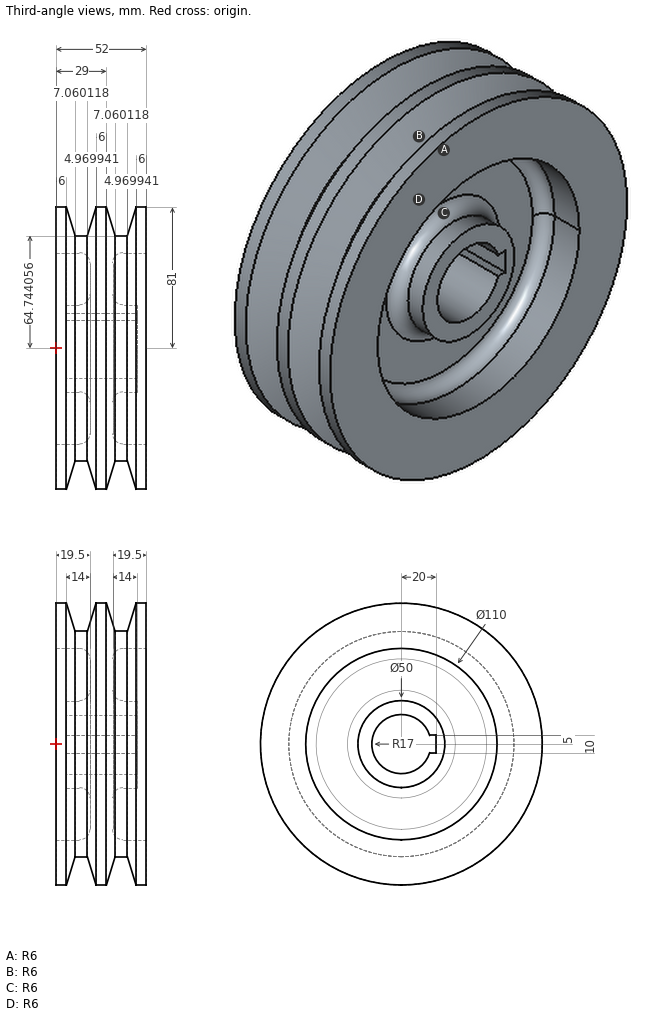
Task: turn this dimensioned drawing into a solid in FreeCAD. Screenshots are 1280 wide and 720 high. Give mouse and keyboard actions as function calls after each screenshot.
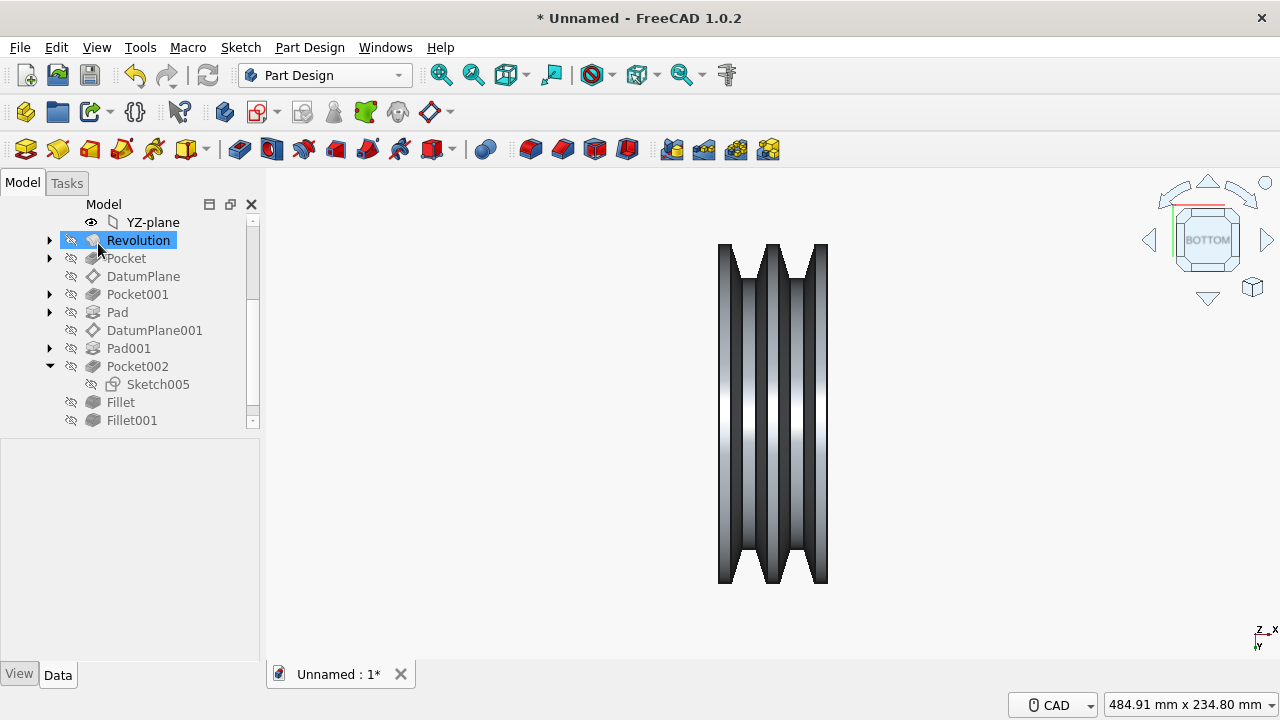
key(4)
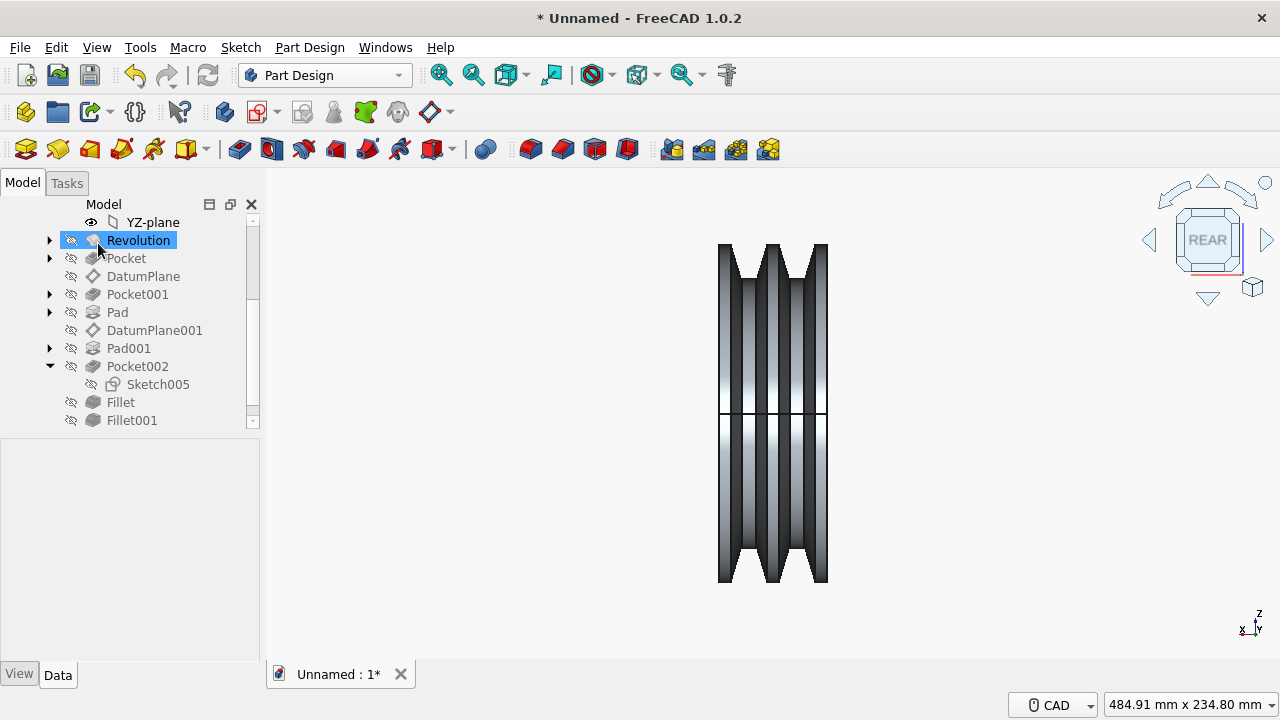
key(6)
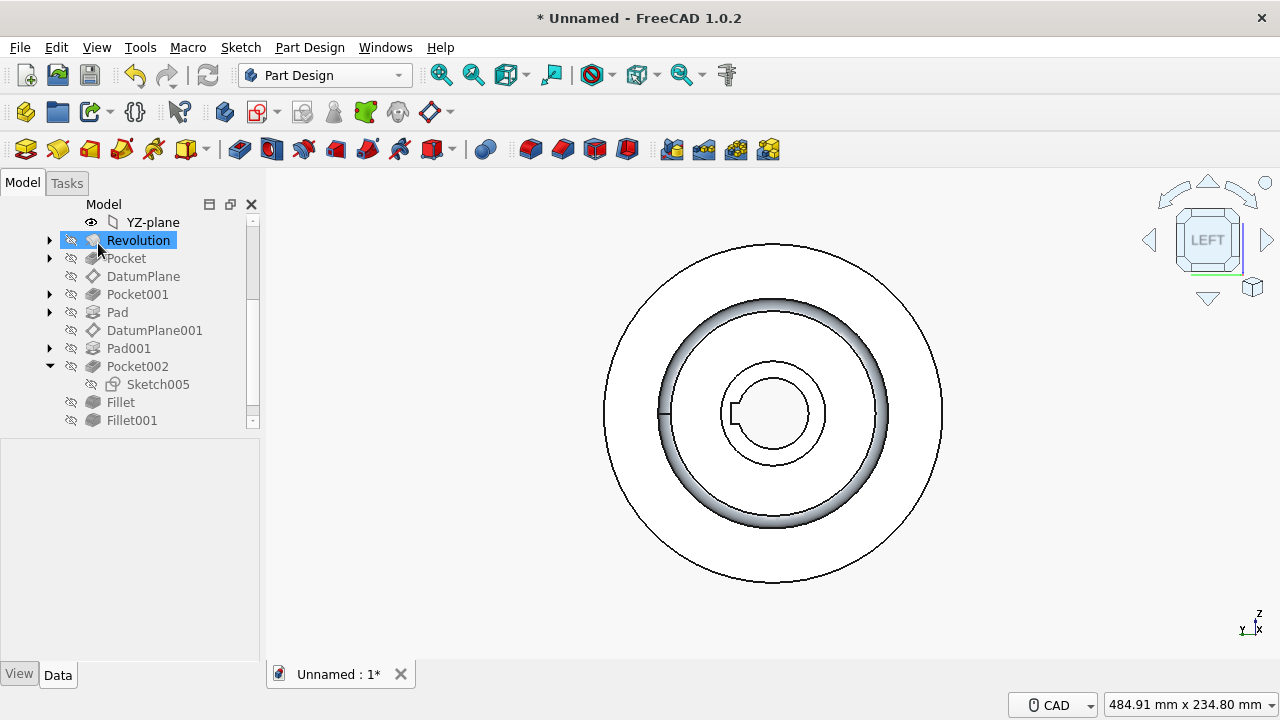
key(v)
key(3)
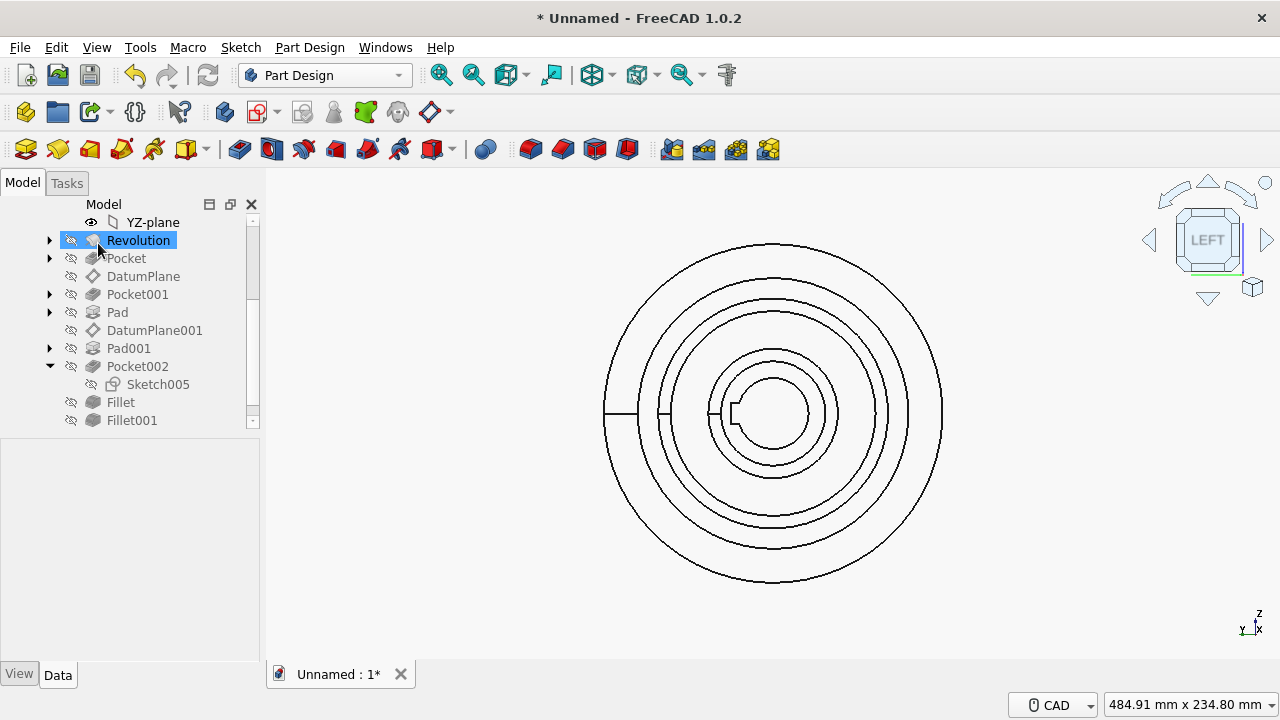
key(0)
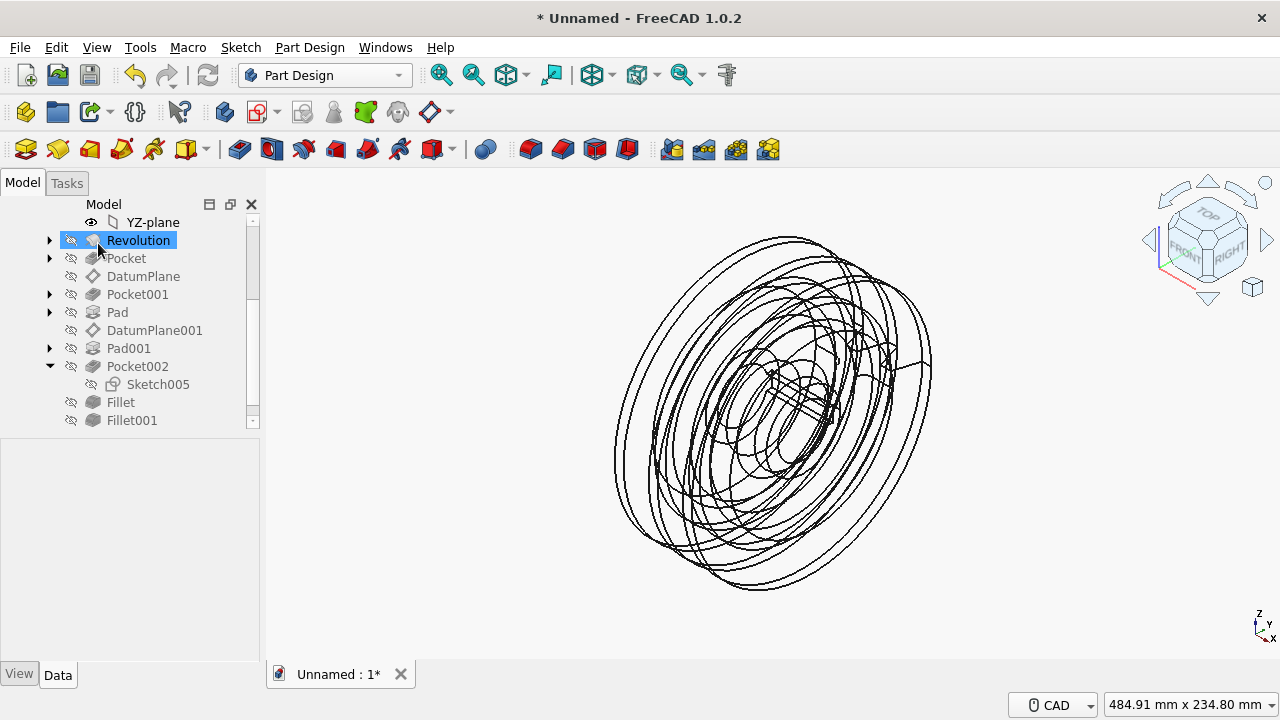
click(726, 428)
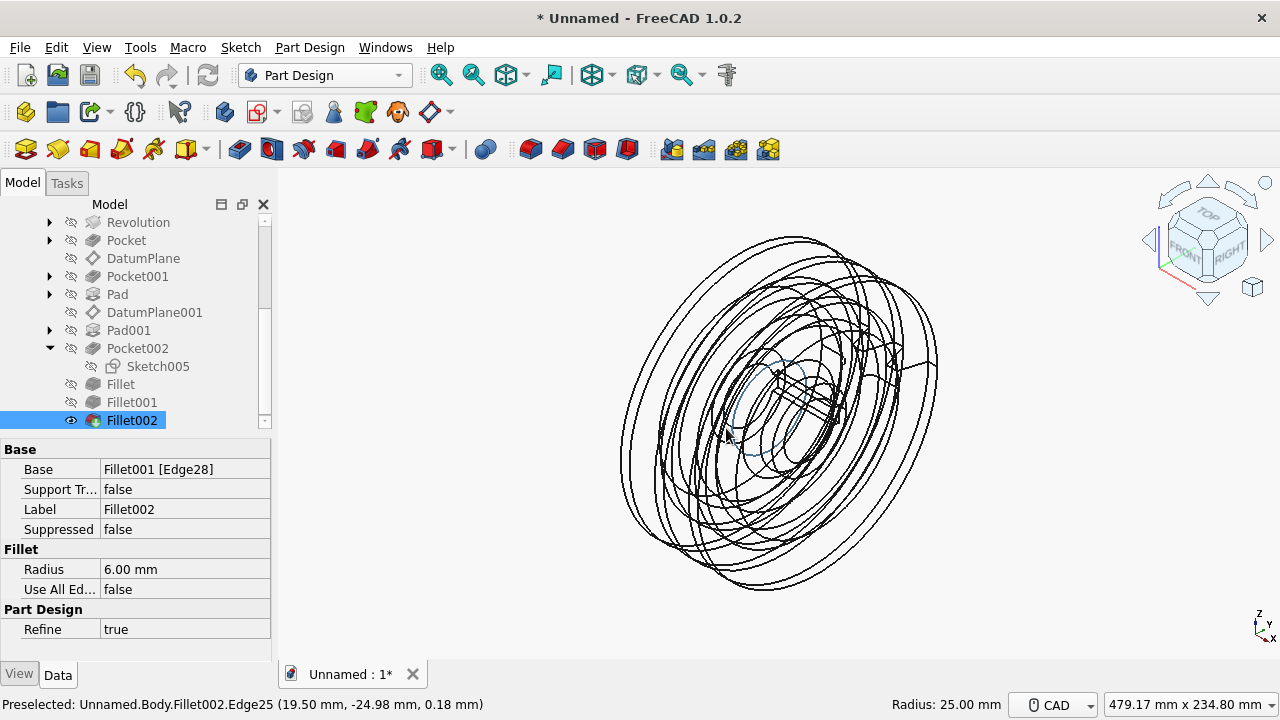
key(v)
key(1)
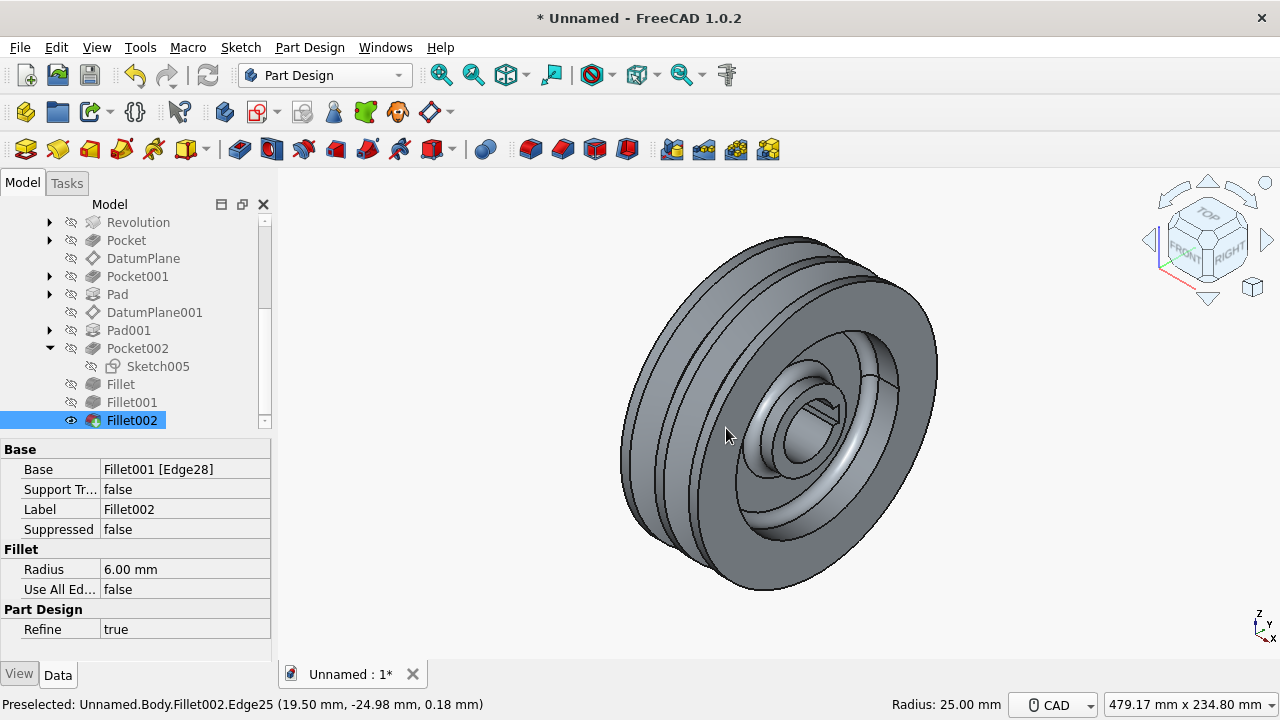
click(532, 150)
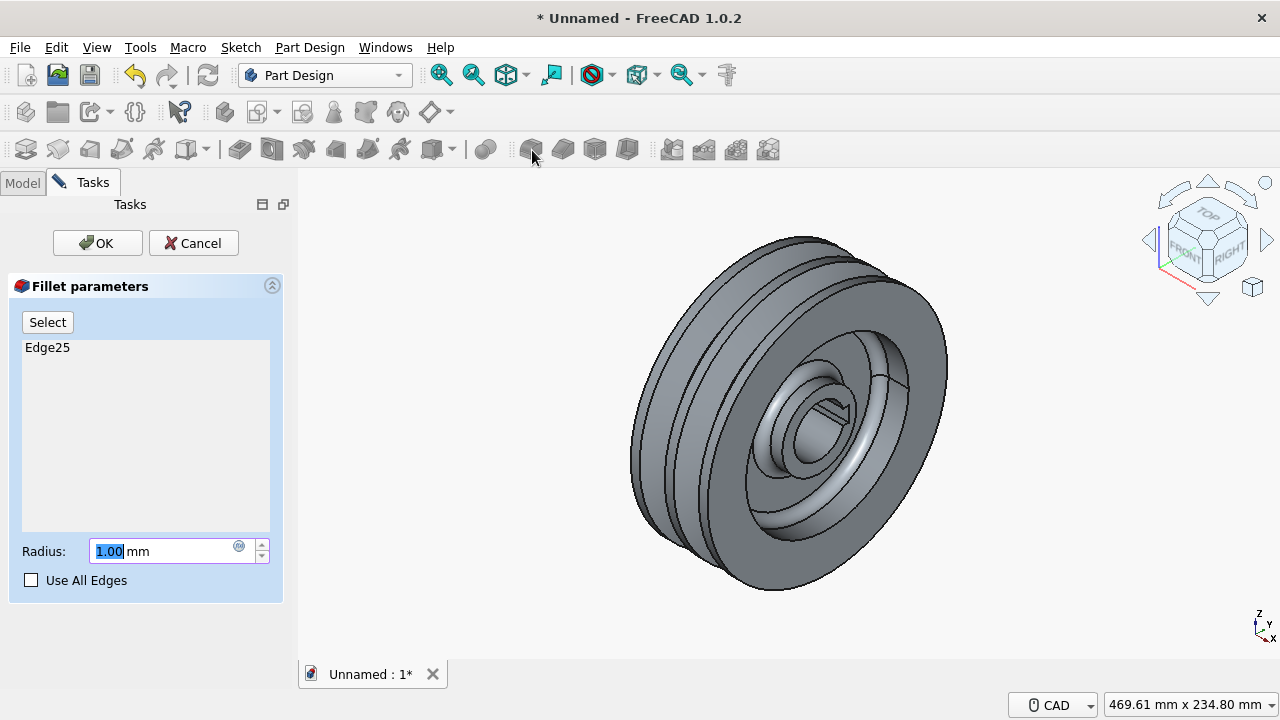
text(6)
key(Tab)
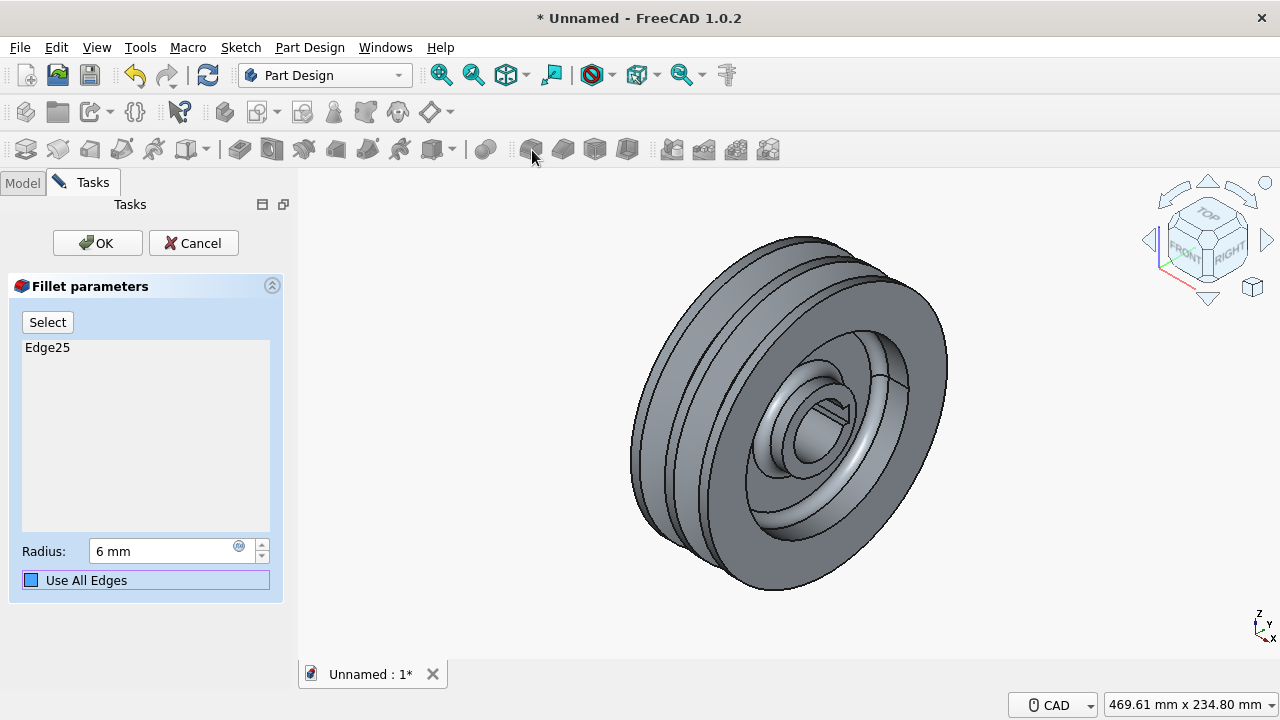
click(98, 243)